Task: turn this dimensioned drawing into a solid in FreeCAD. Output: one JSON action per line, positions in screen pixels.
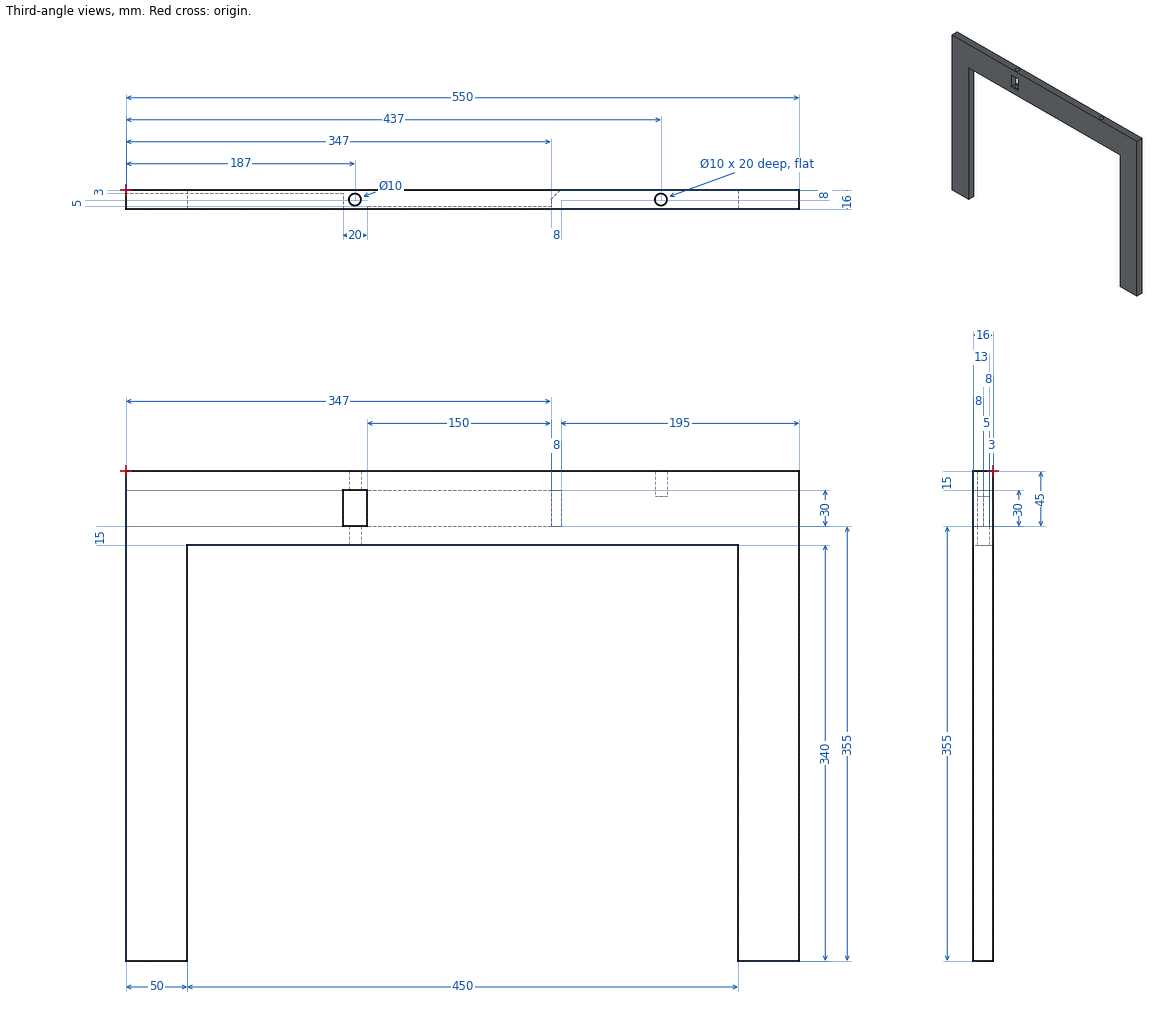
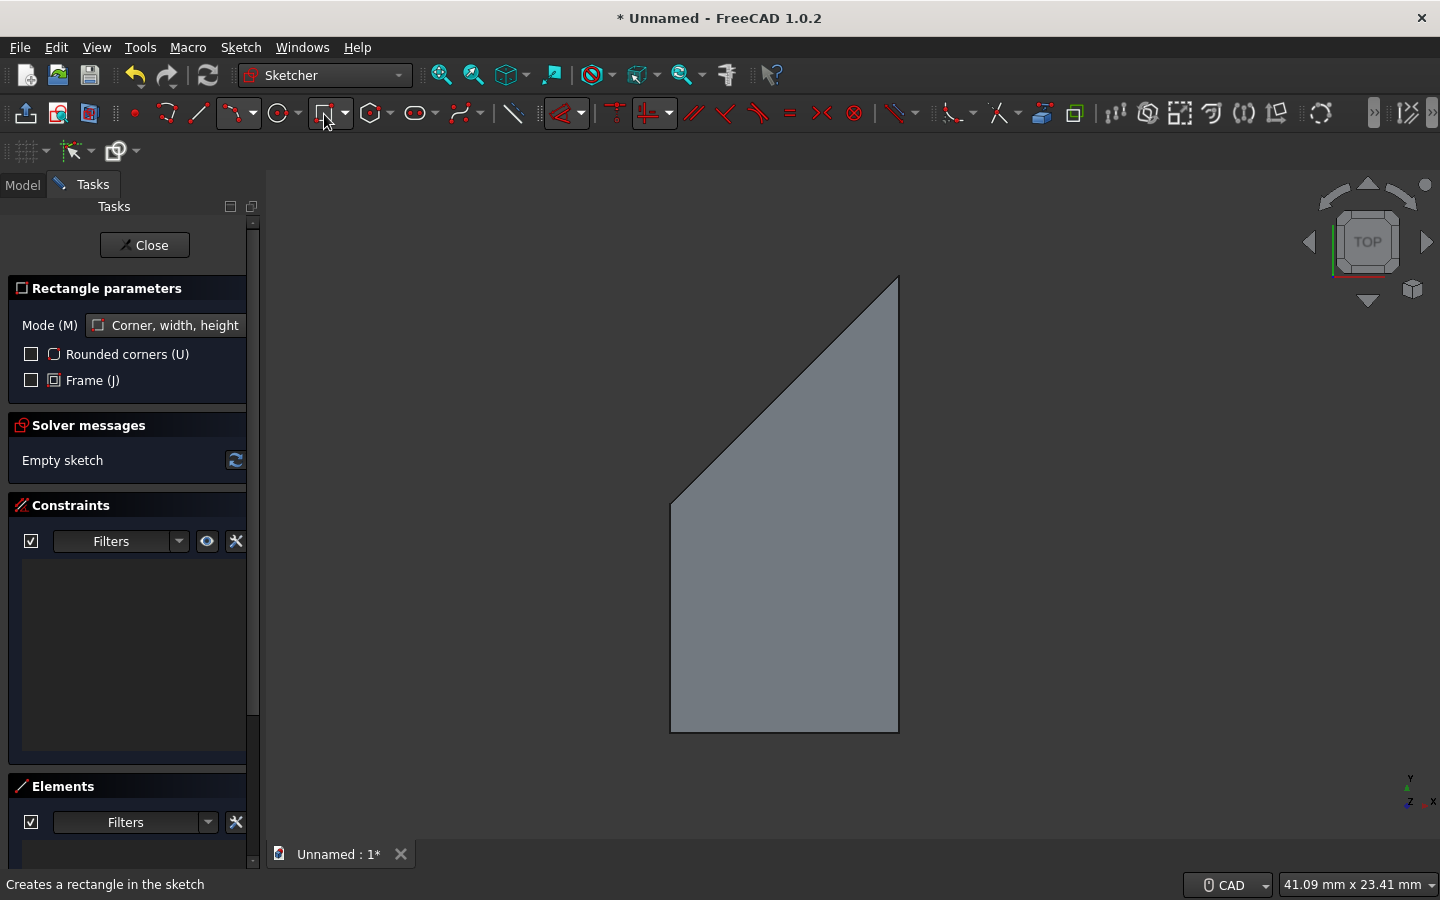
{"action": "left_click", "coordinate": [670, 276]}
{"action": "left_click", "coordinate": [899, 733]}
{"action": "key", "text": "Escape"}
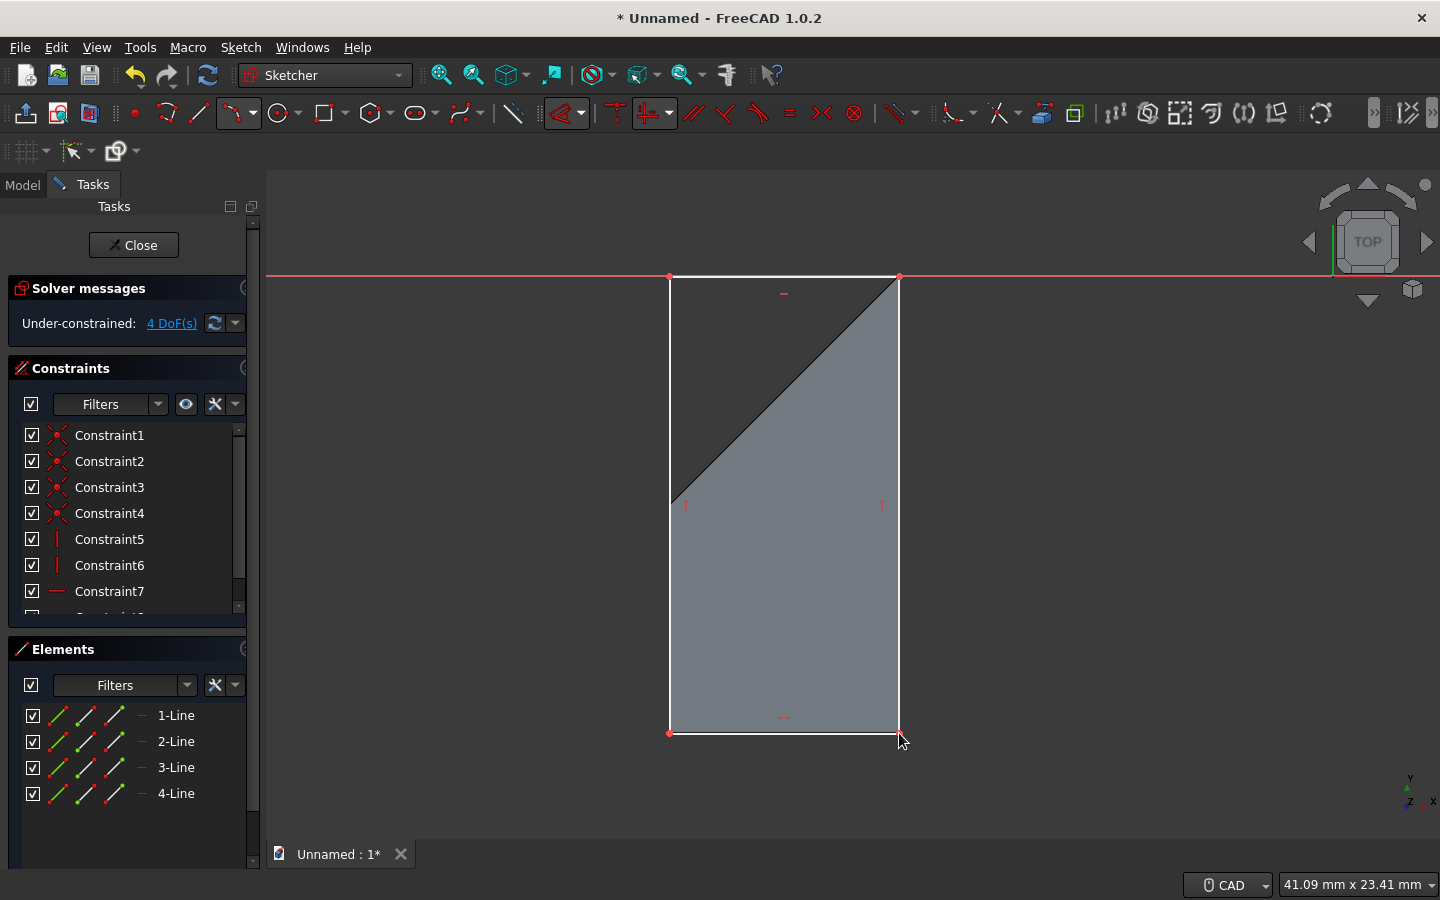
{"action": "left_click", "coordinate": [670, 277]}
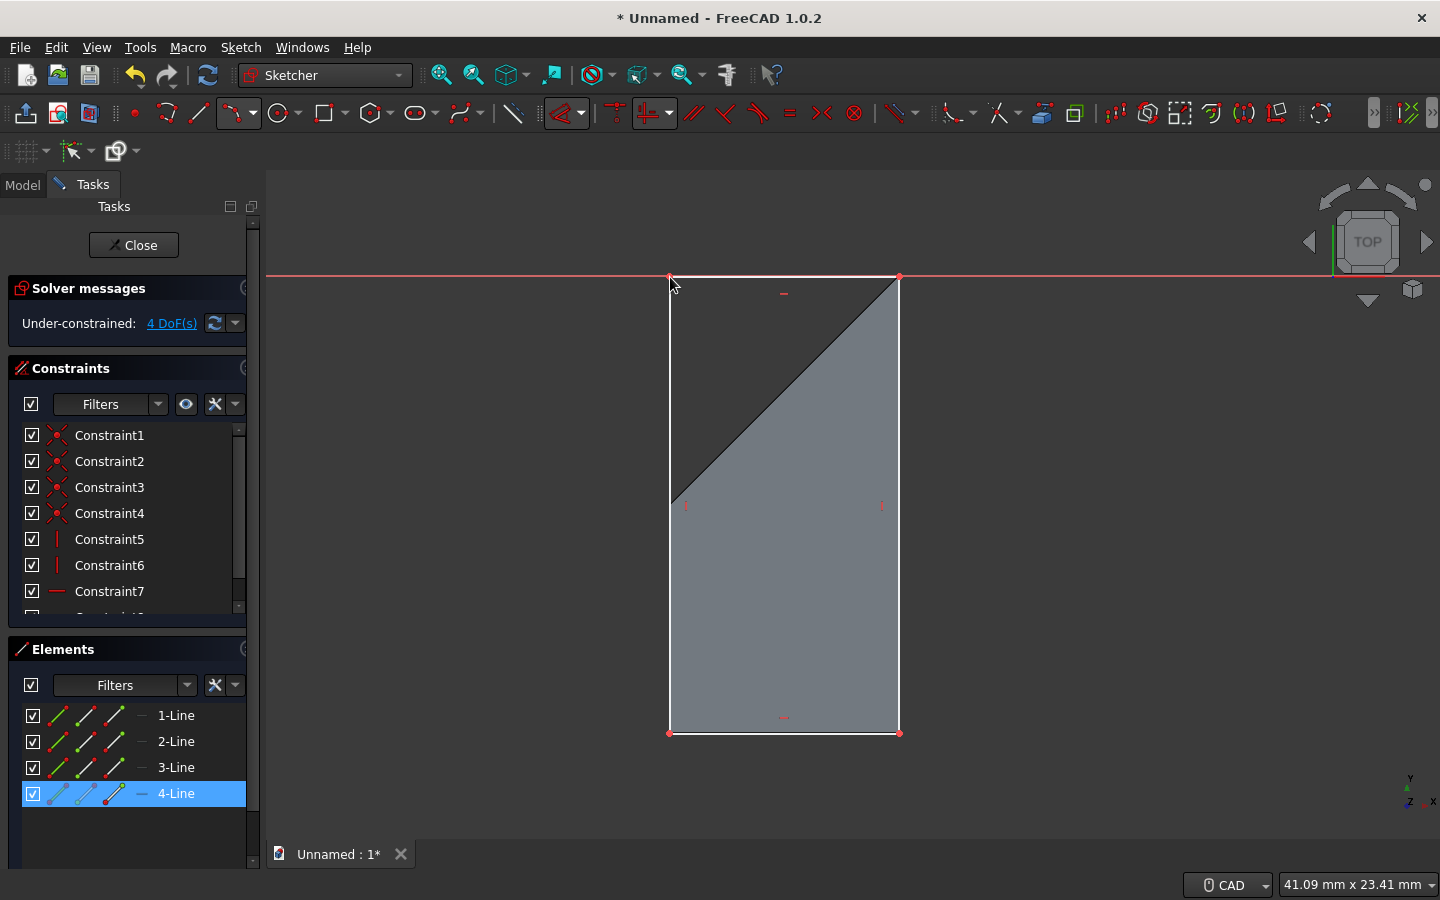
{"action": "left_click", "coordinate": [364, 276]}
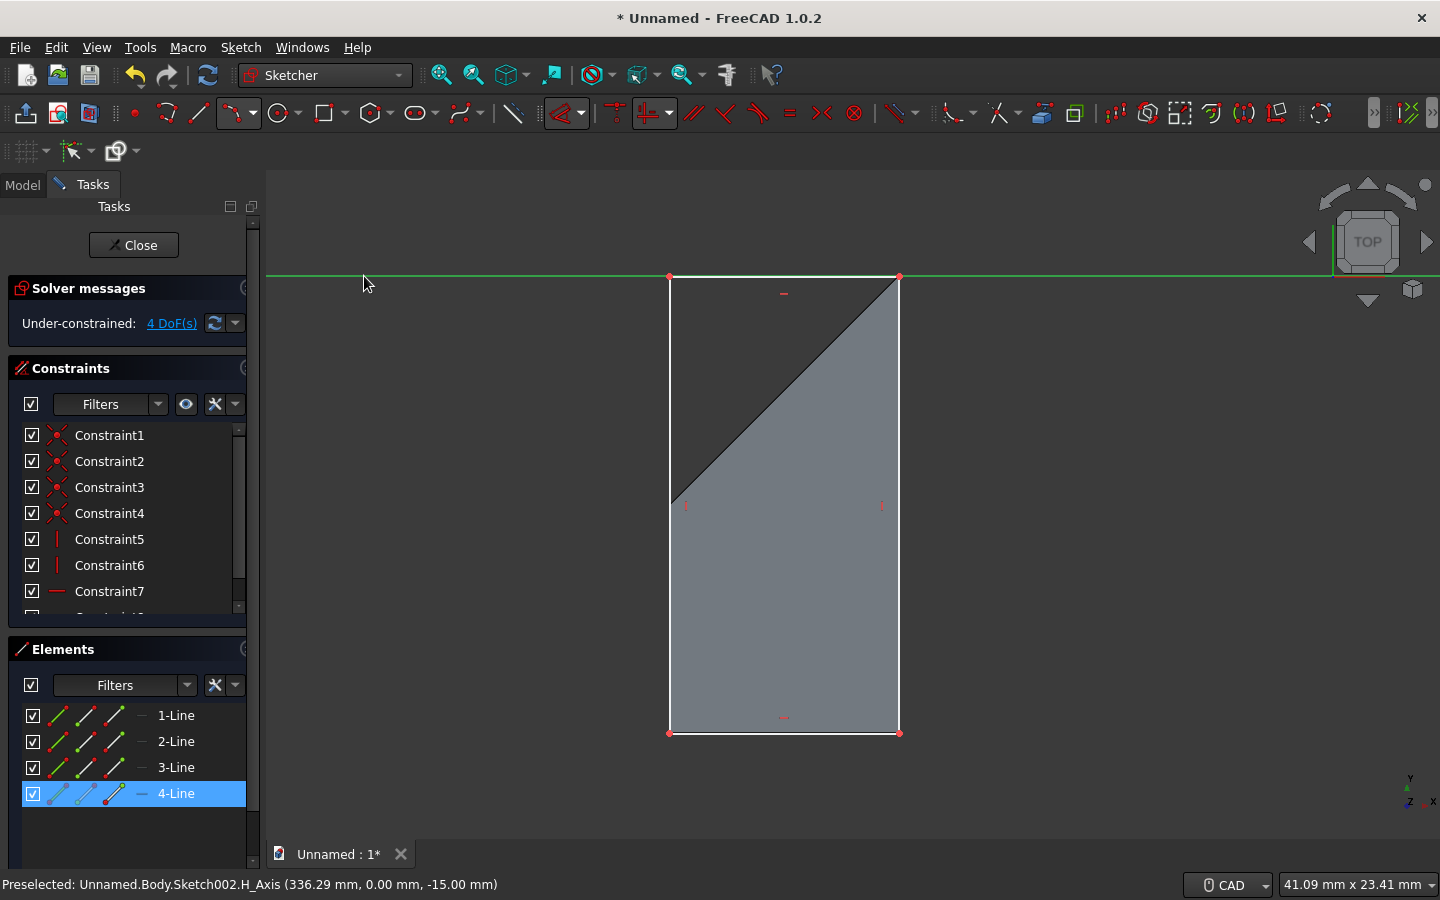
{"action": "left_click", "coordinate": [616, 114]}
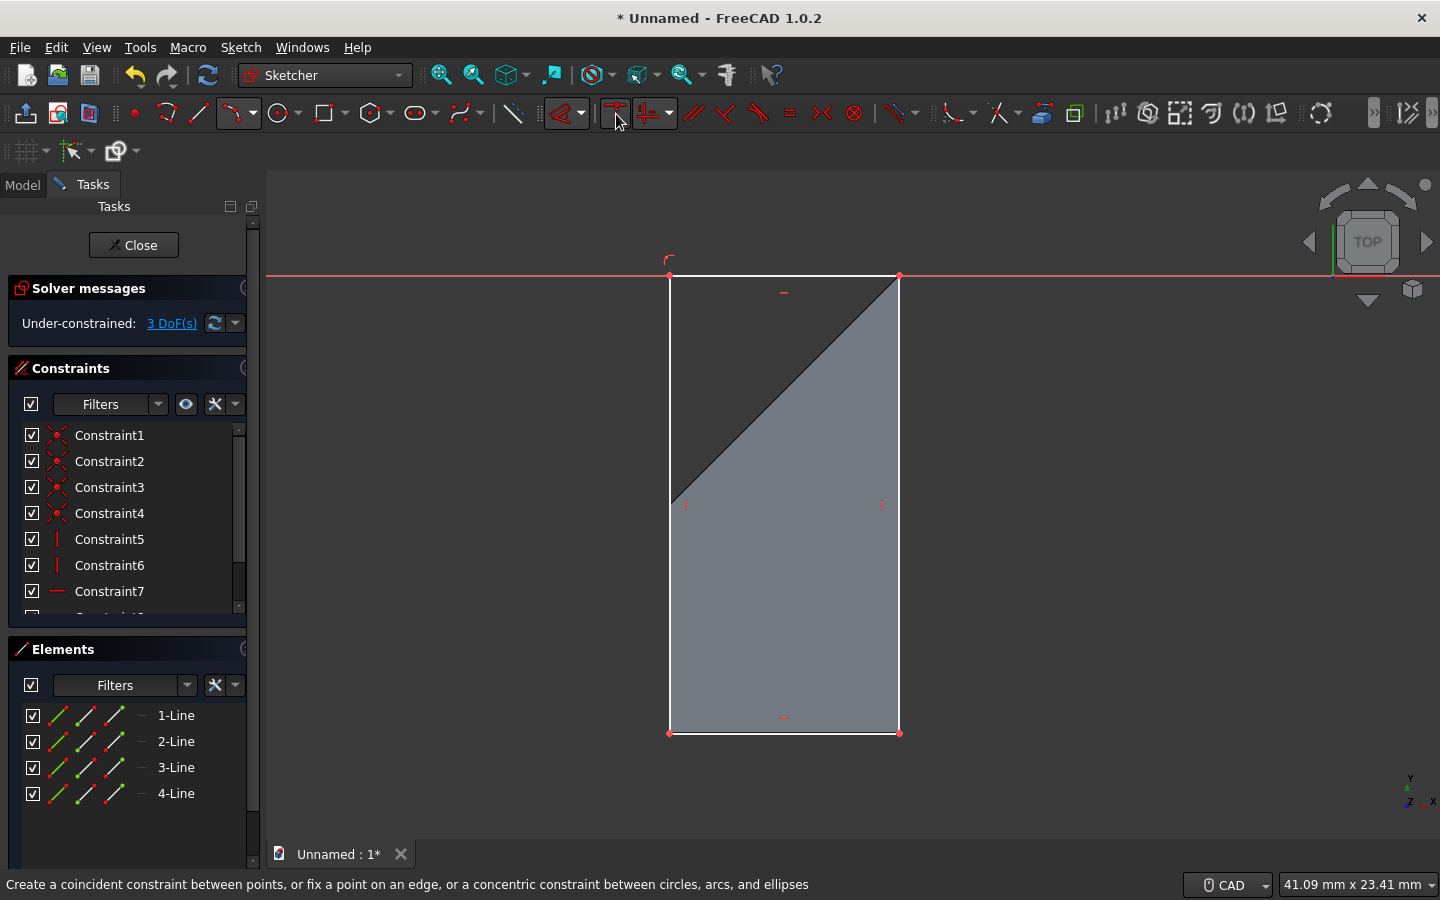
{"action": "left_click", "coordinate": [739, 734]}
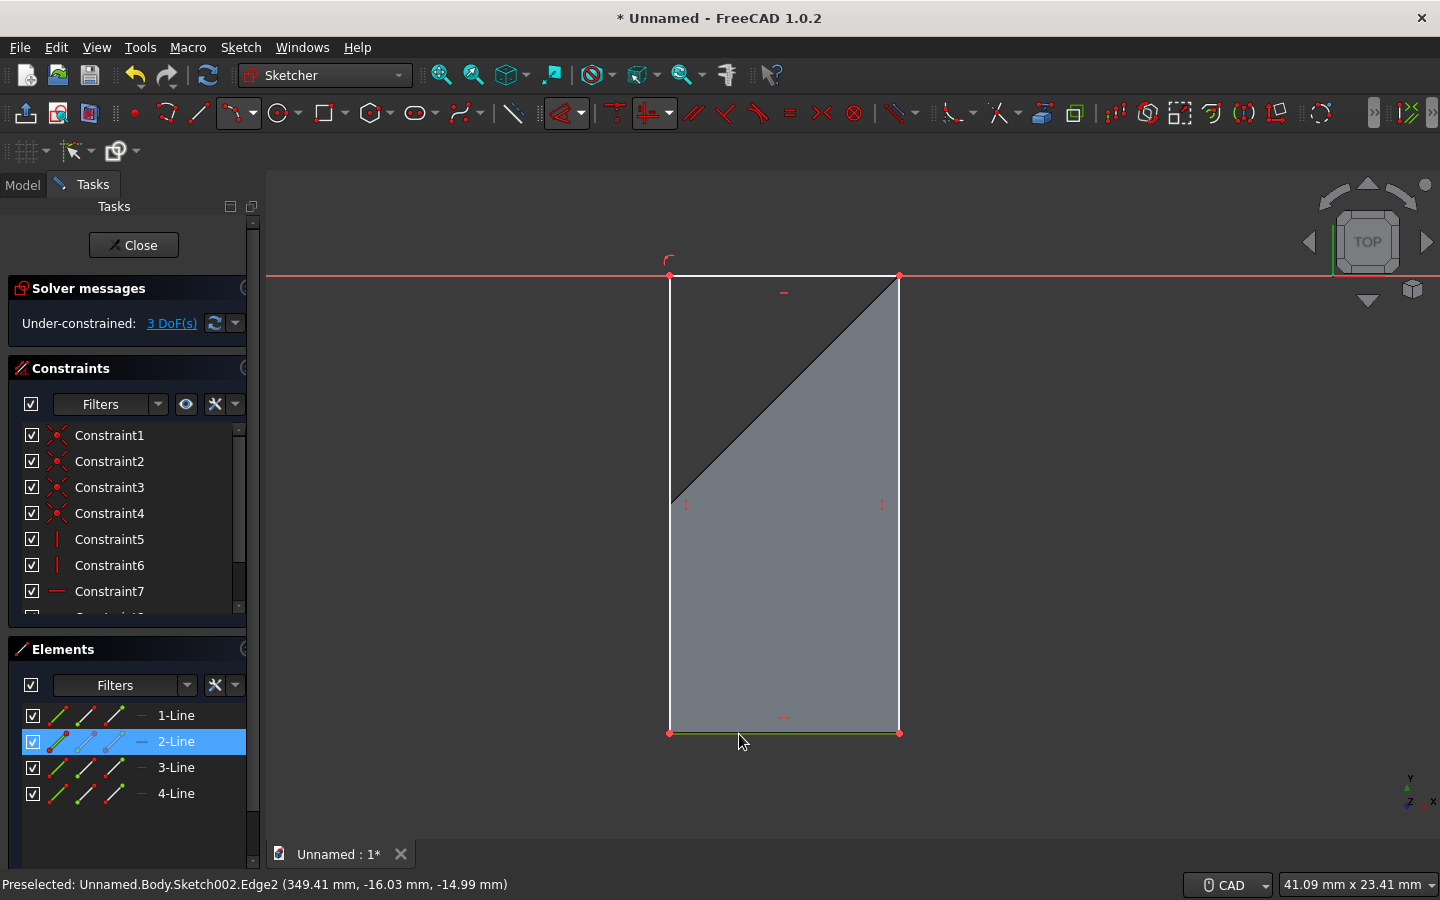
{"action": "key", "text": "l"}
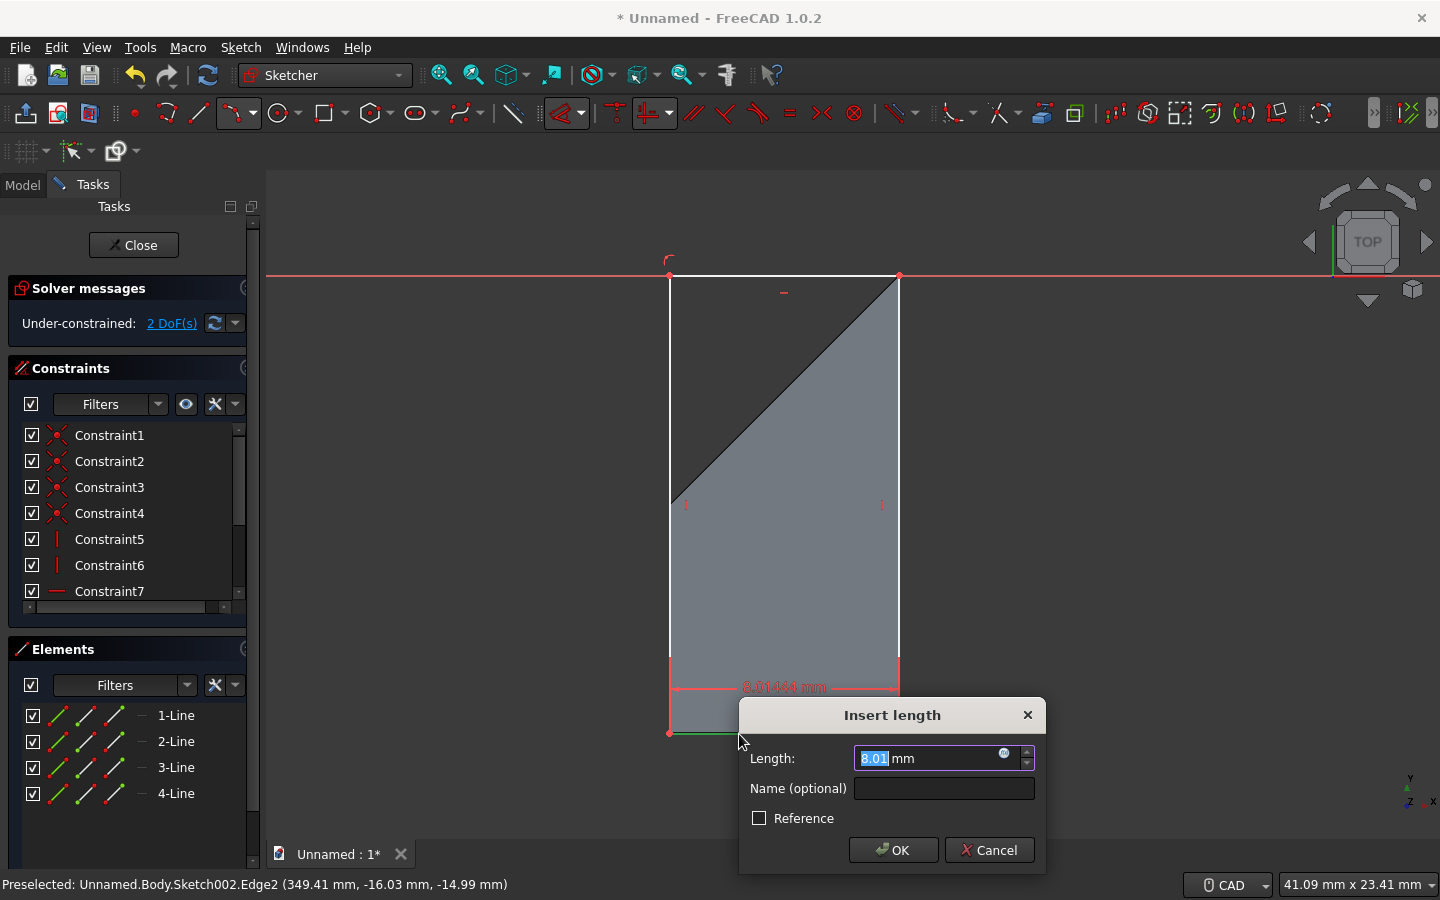
{"action": "type", "text": "8"}
{"action": "key", "text": "Return"}